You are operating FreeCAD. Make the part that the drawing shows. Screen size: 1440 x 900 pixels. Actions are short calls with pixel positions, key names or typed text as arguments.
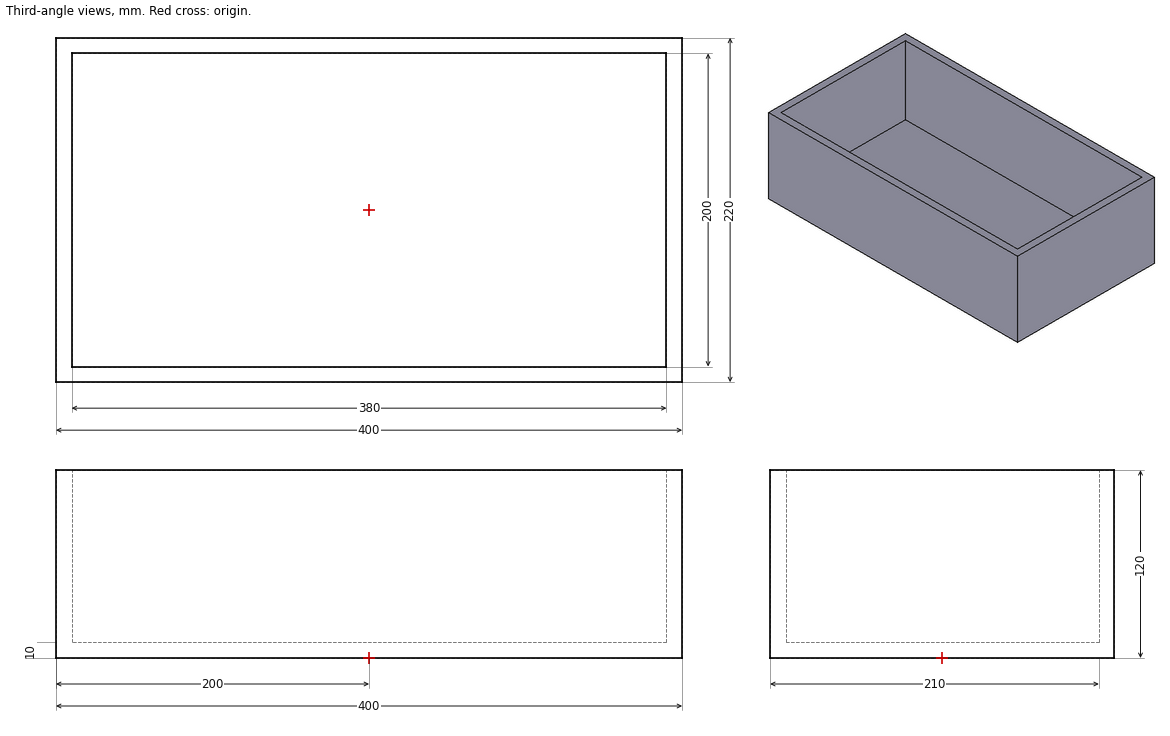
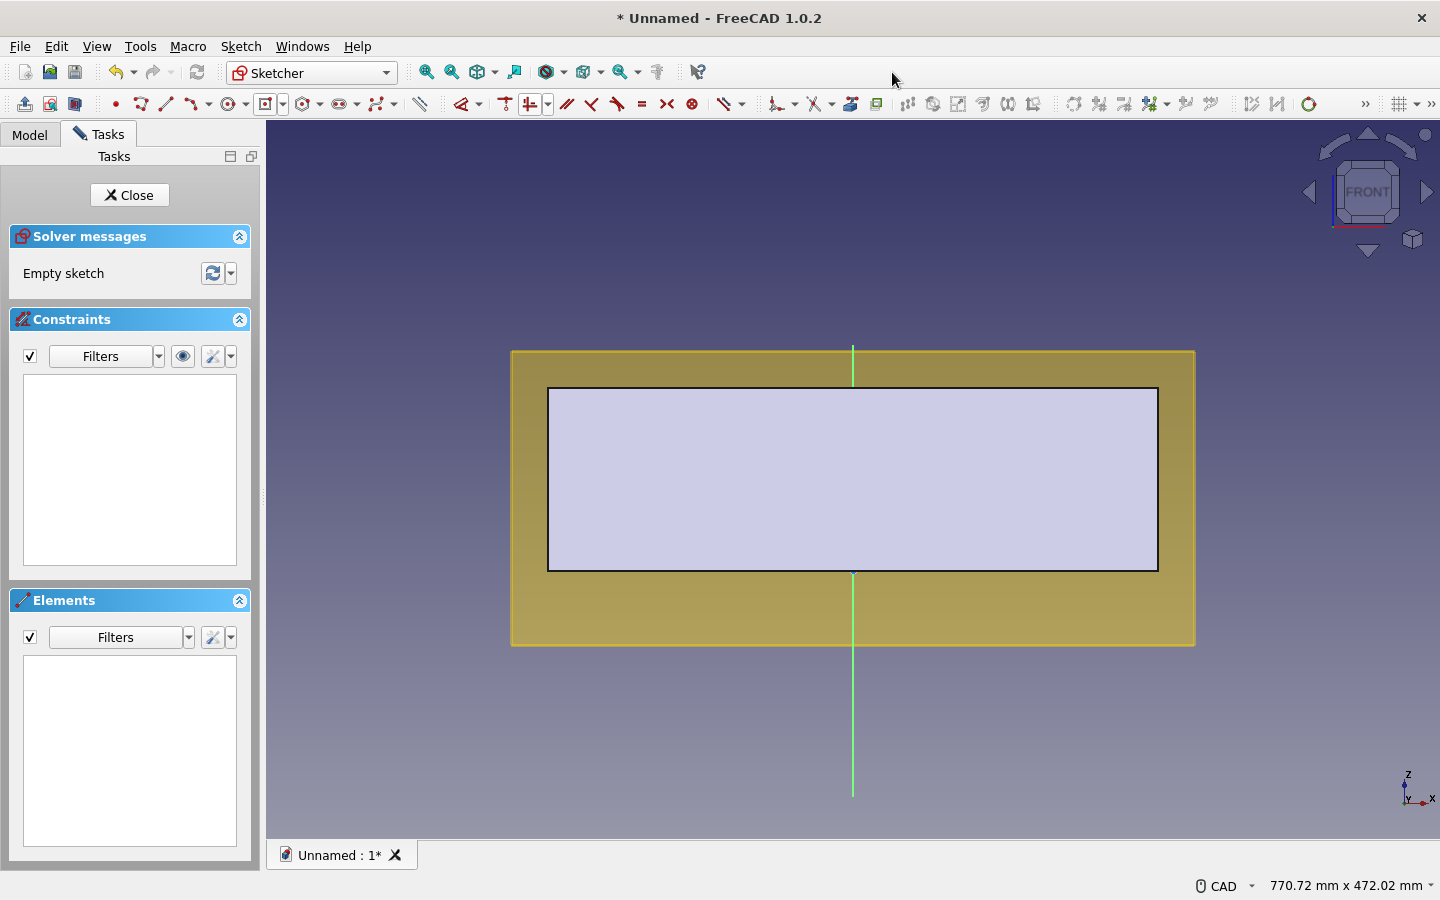
click(75, 104)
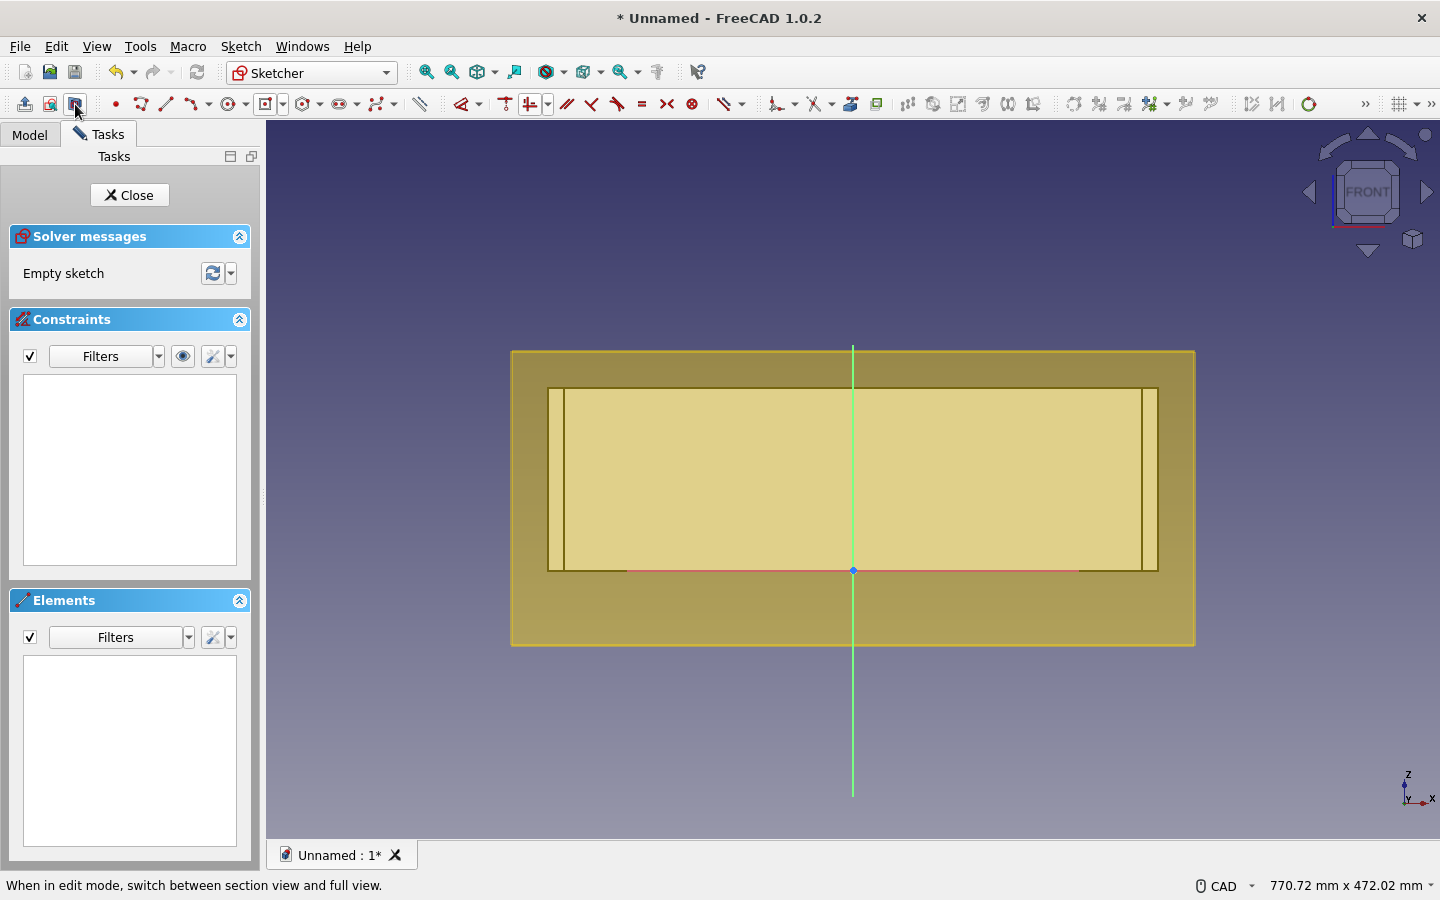
key(g)
key(r)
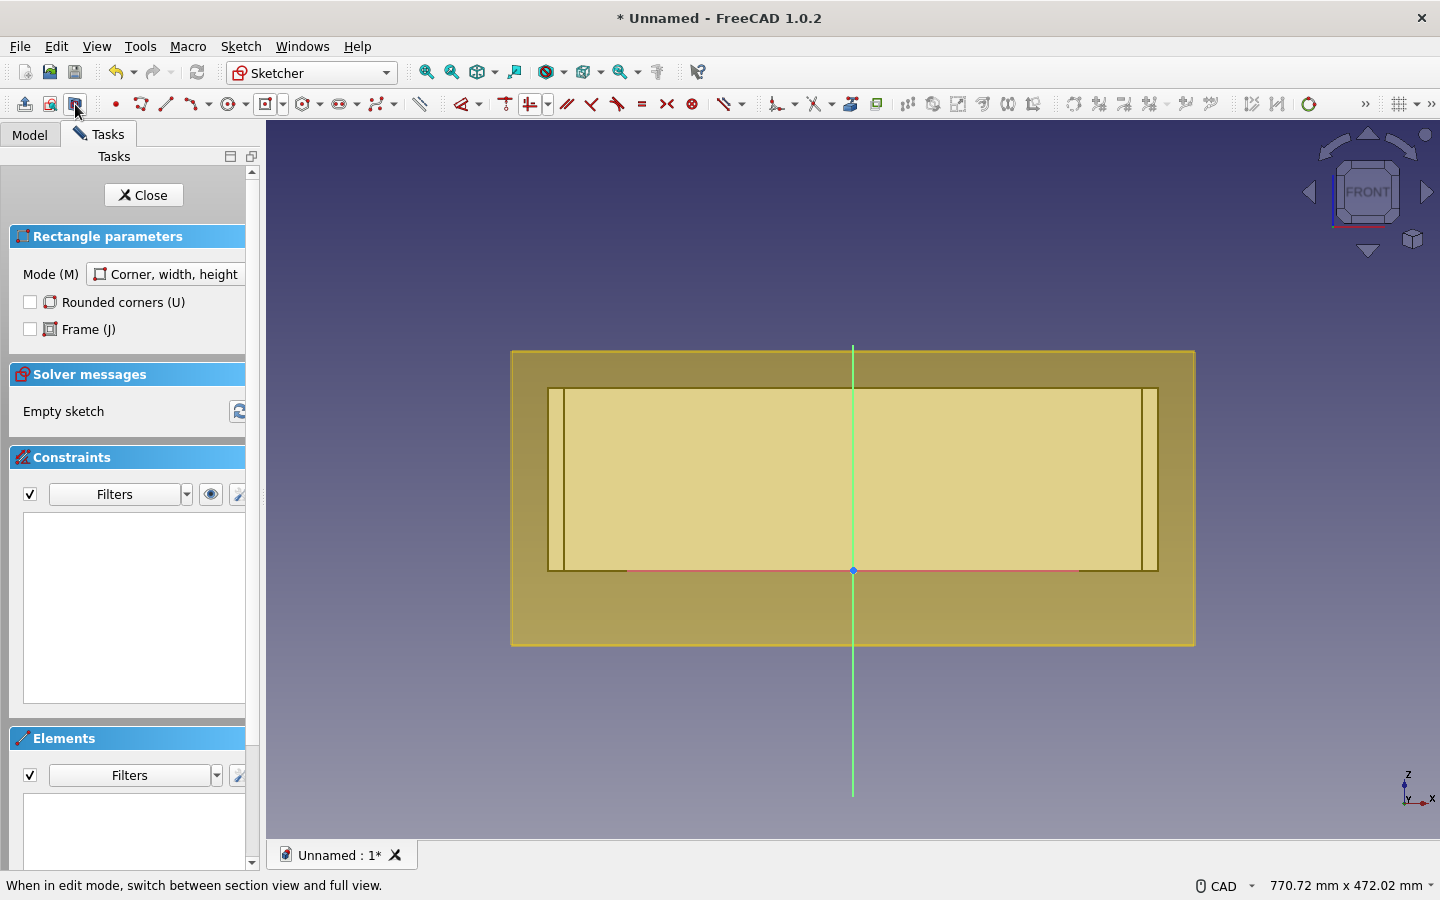
click(548, 556)
click(1158, 571)
key(Escape)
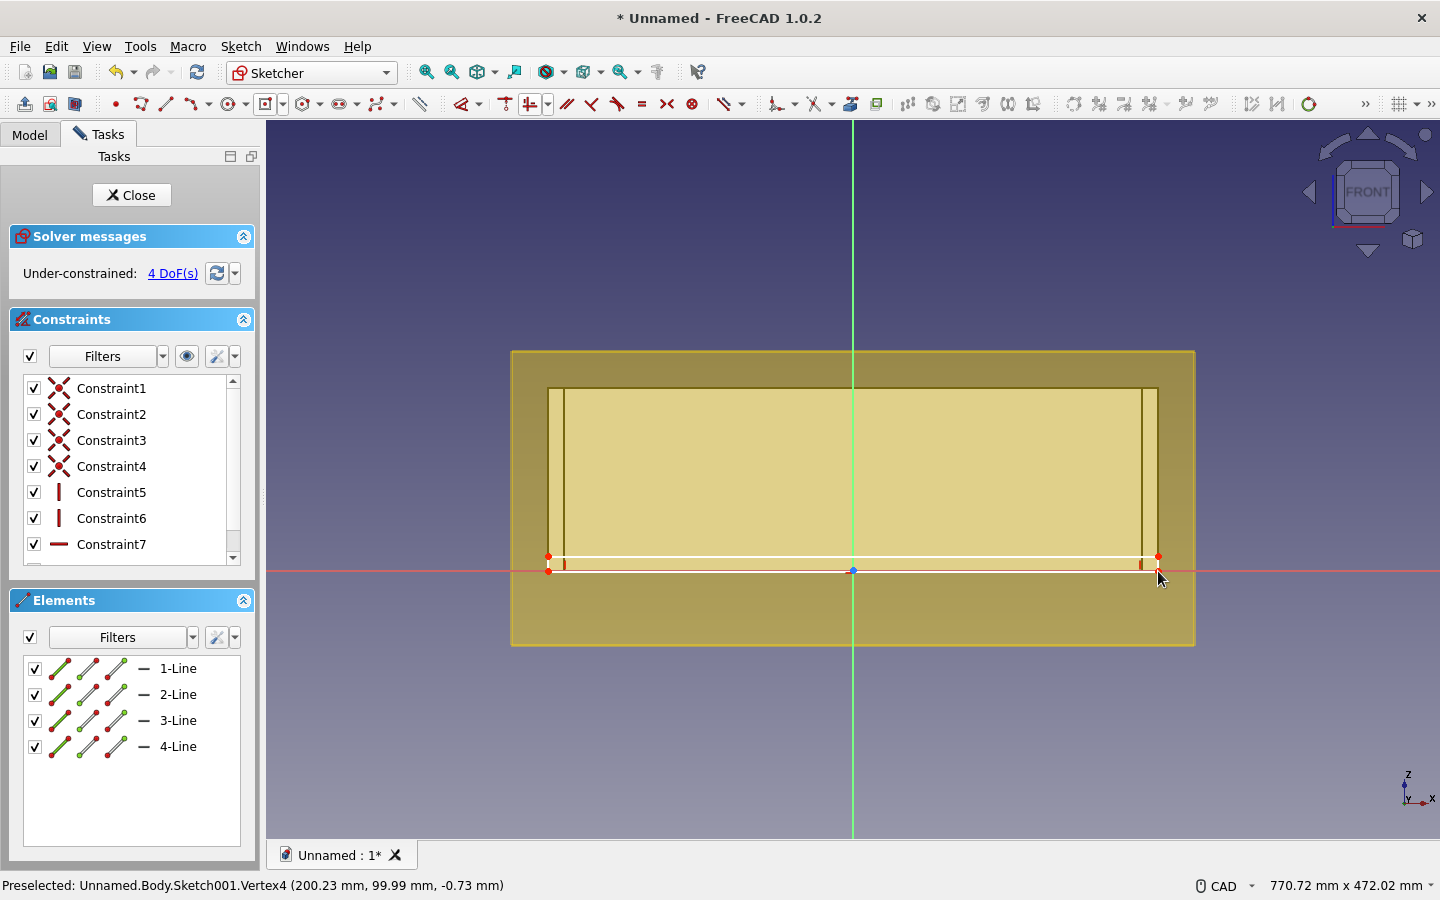
click(548, 572)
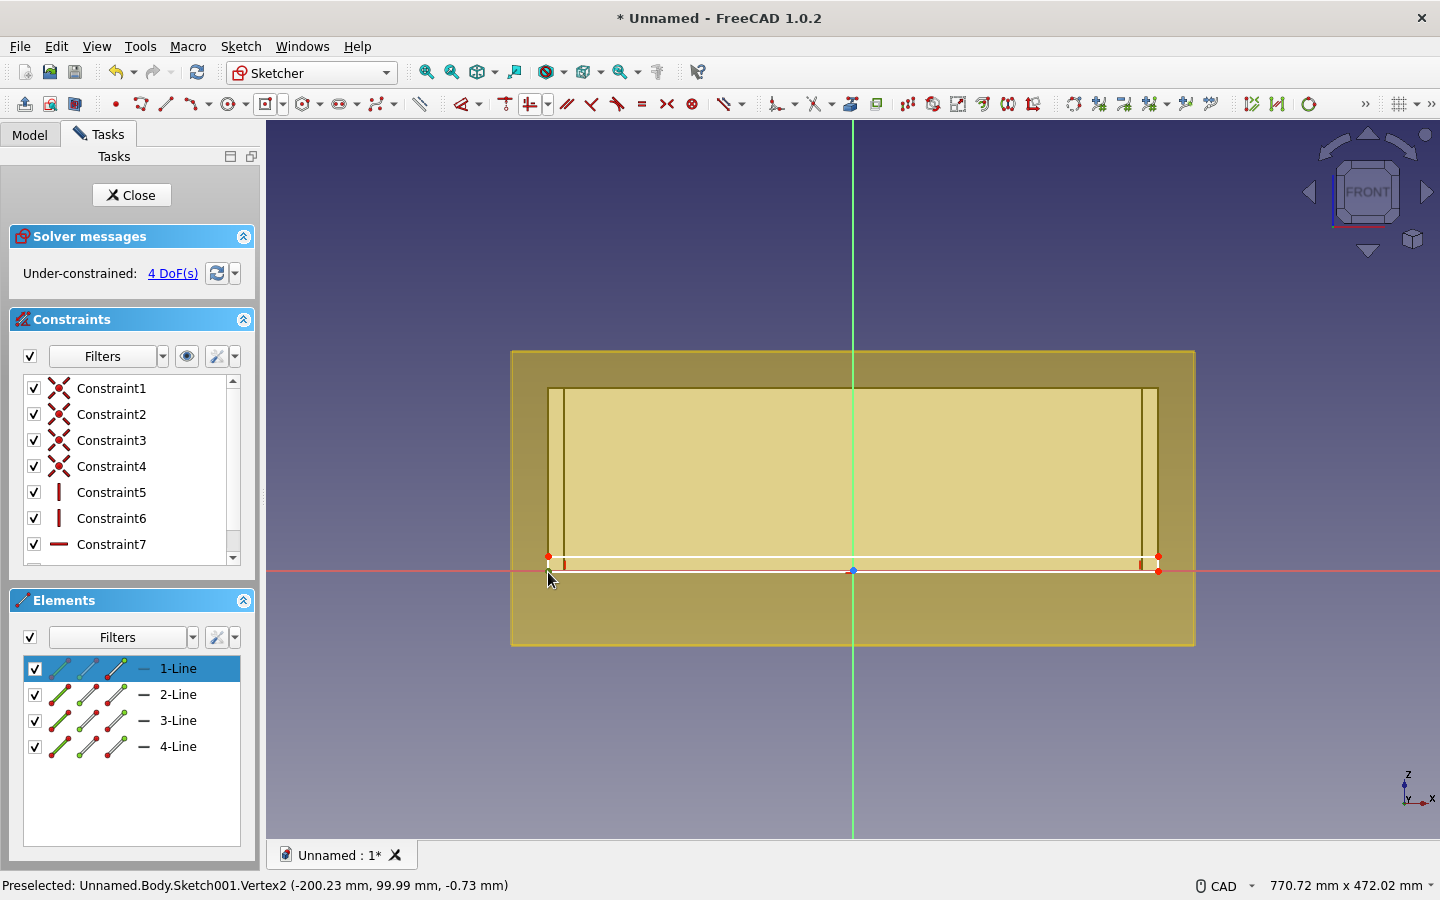
click(364, 571)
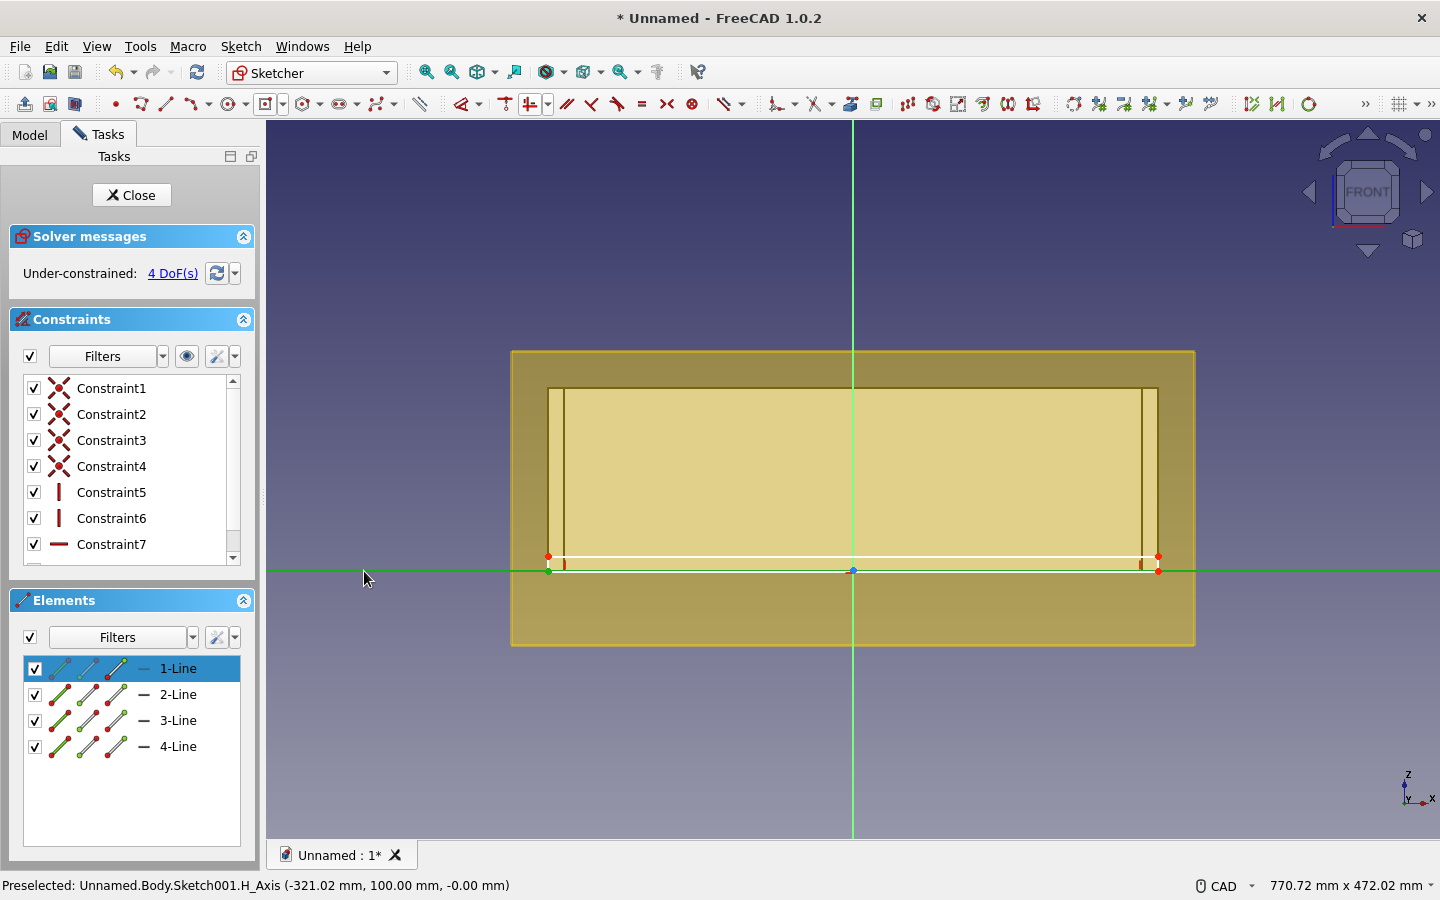
click(505, 104)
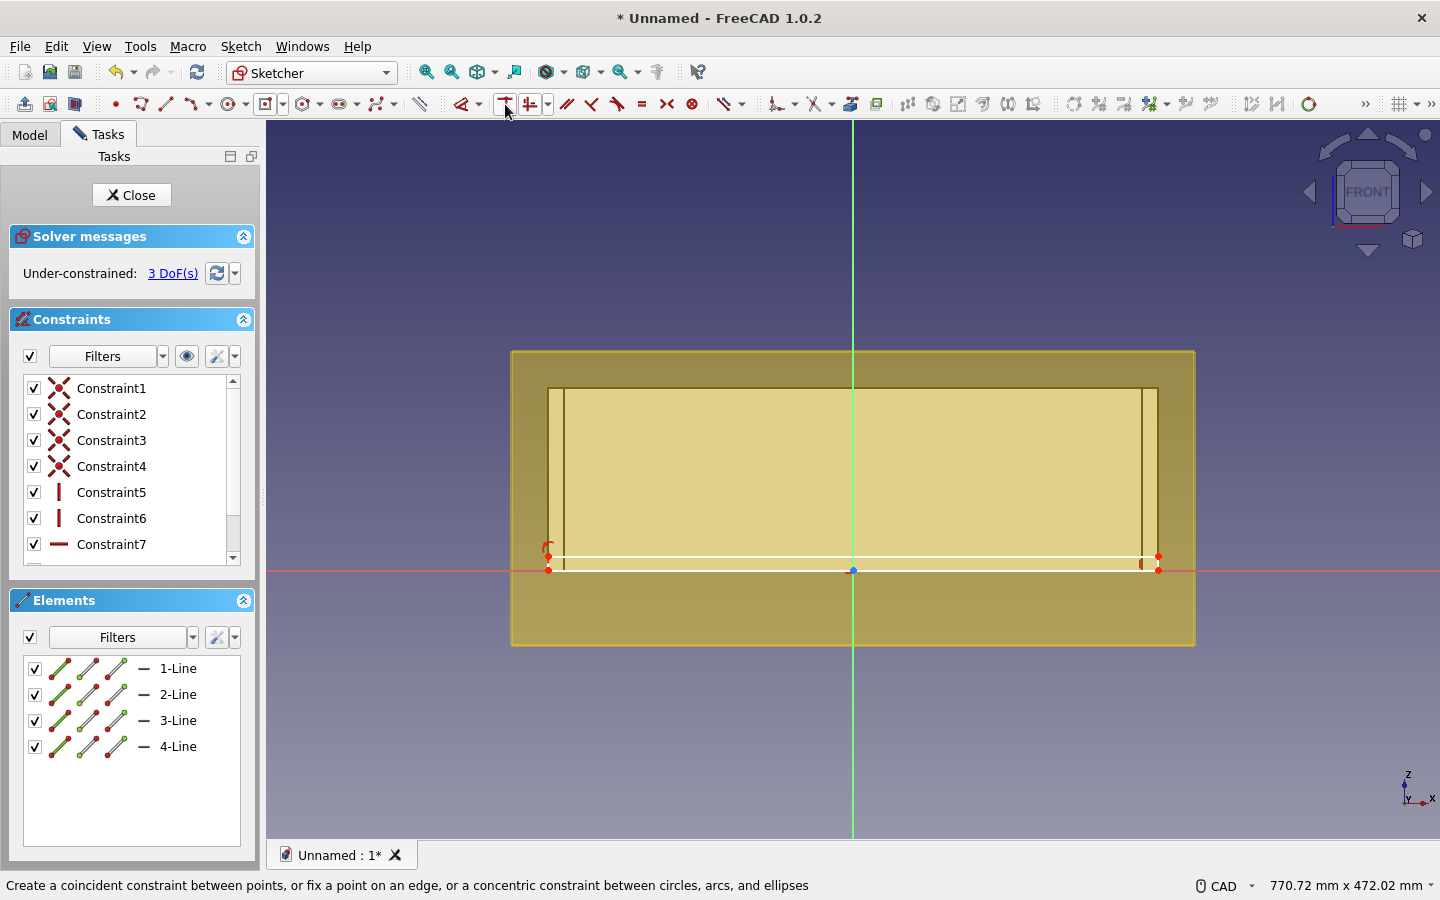
click(460, 104)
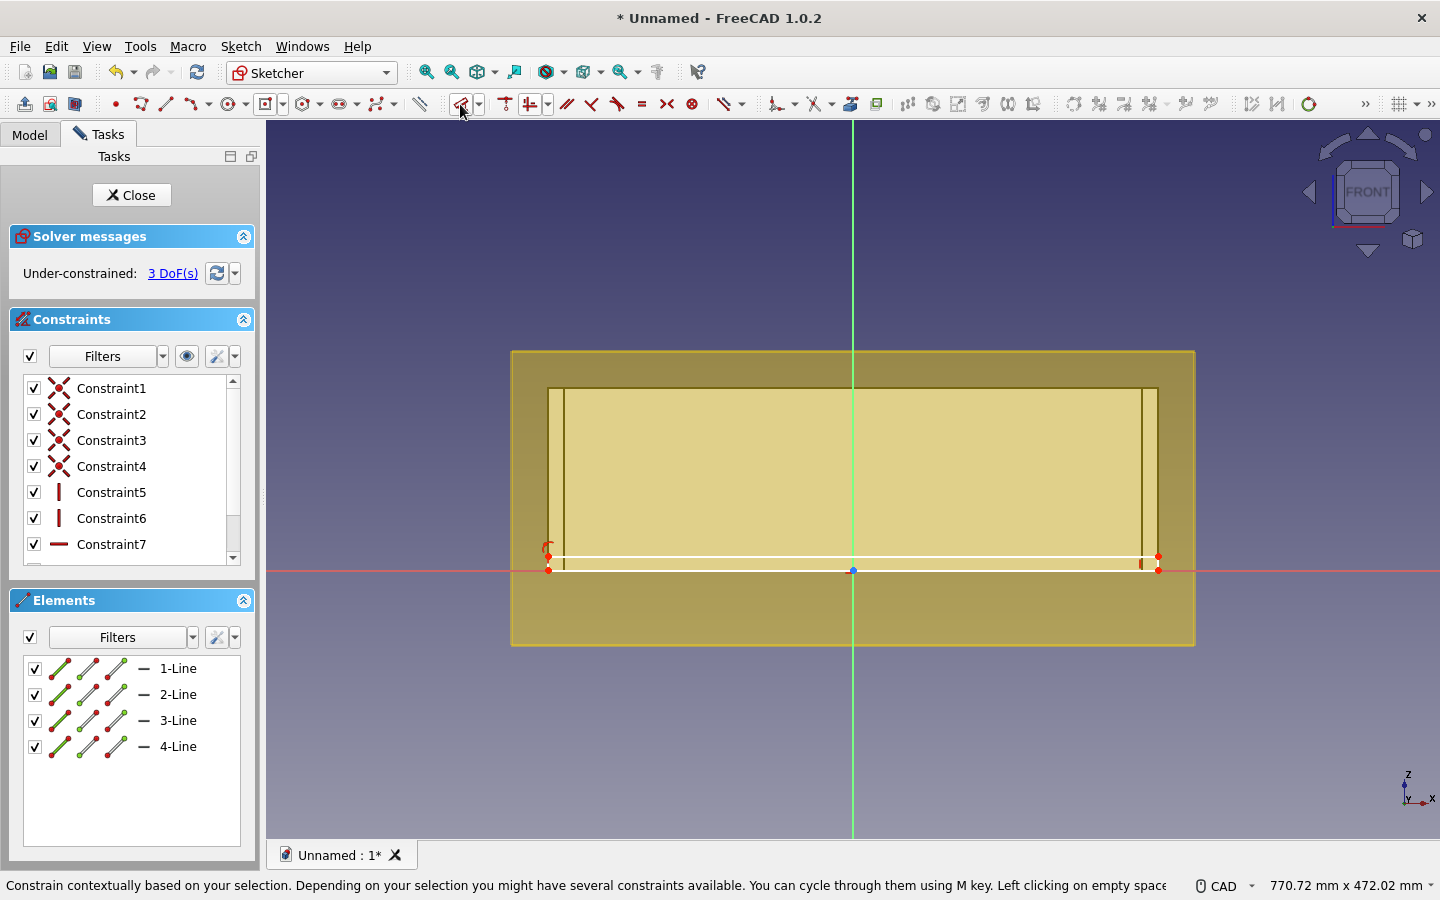
scroll(548, 564, up, 5)